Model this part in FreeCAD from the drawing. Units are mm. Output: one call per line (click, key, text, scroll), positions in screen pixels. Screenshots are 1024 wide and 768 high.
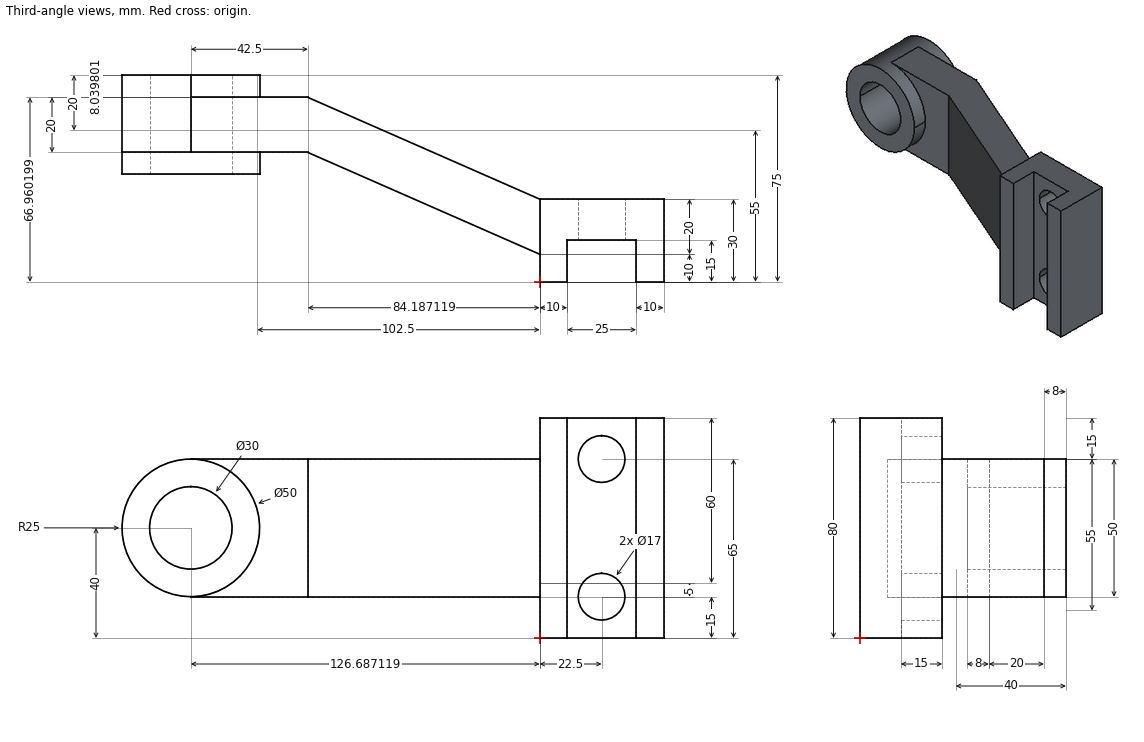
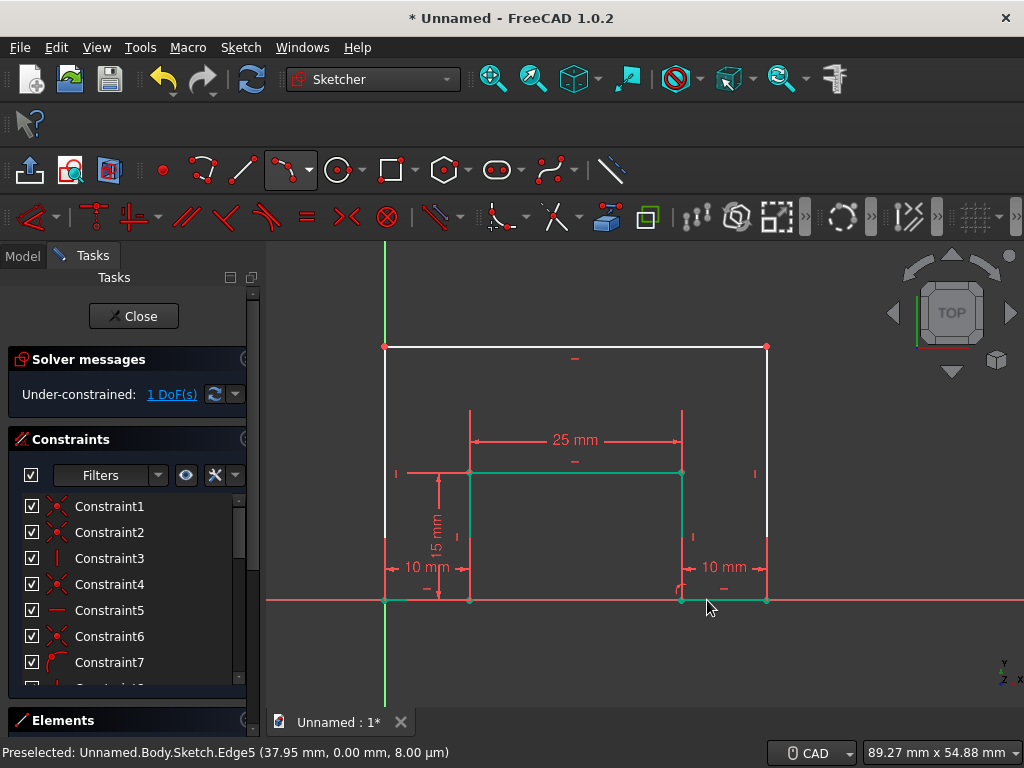
click(767, 524)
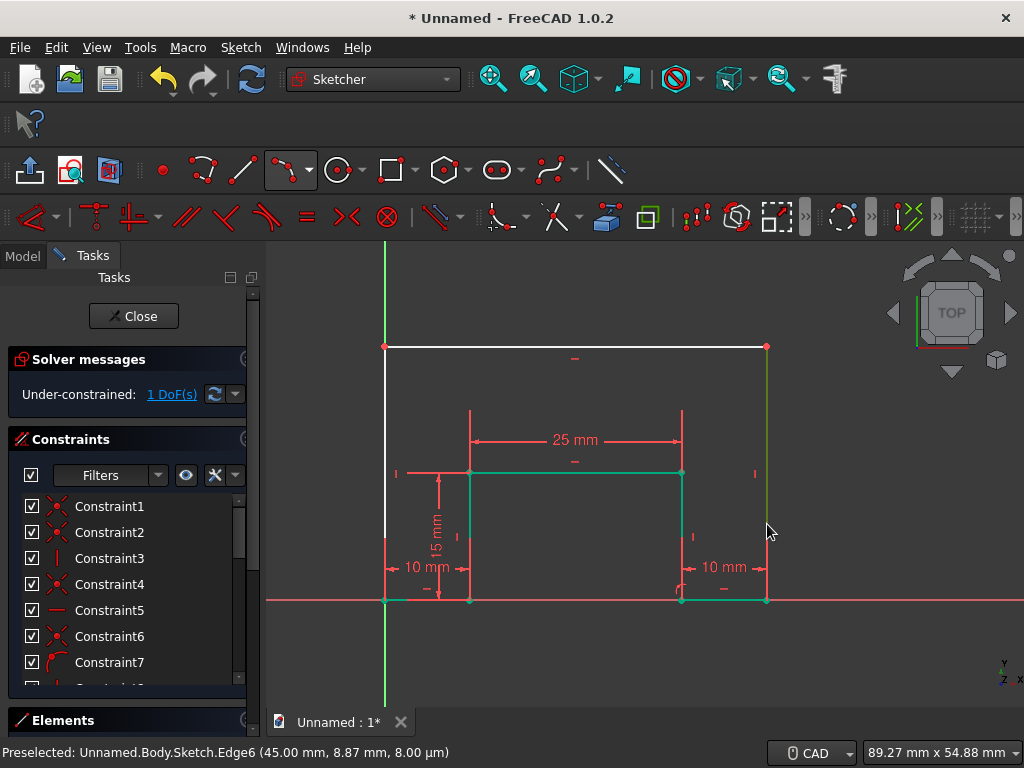
click(58, 218)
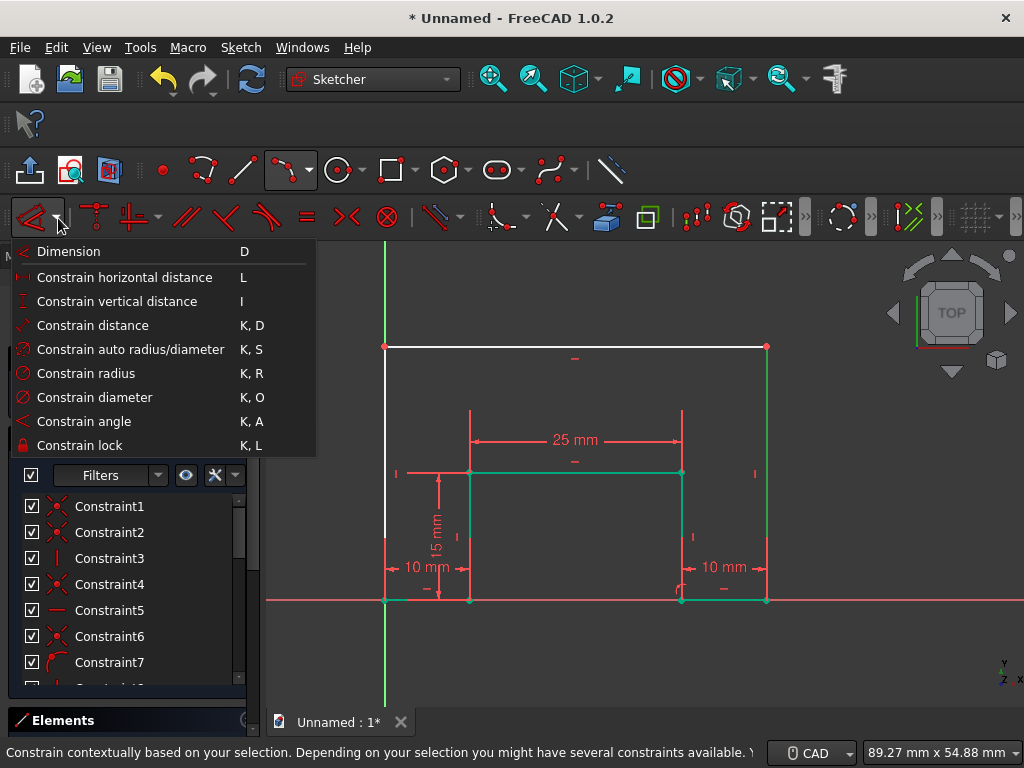
click(164, 301)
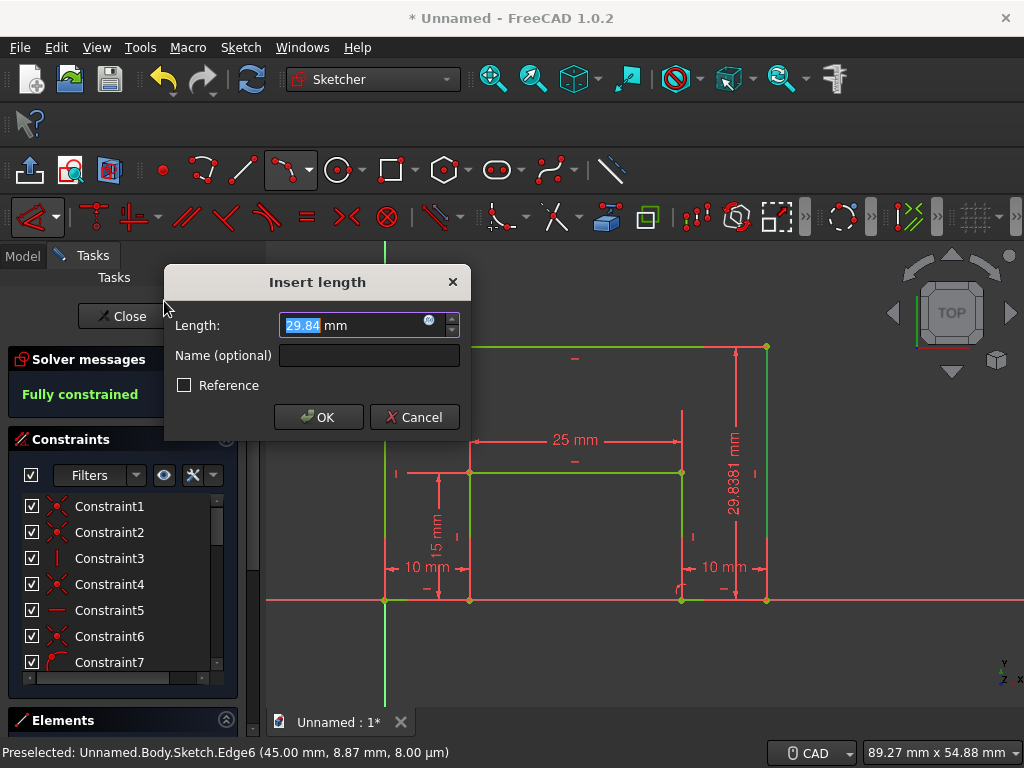
text(30)
key(Return)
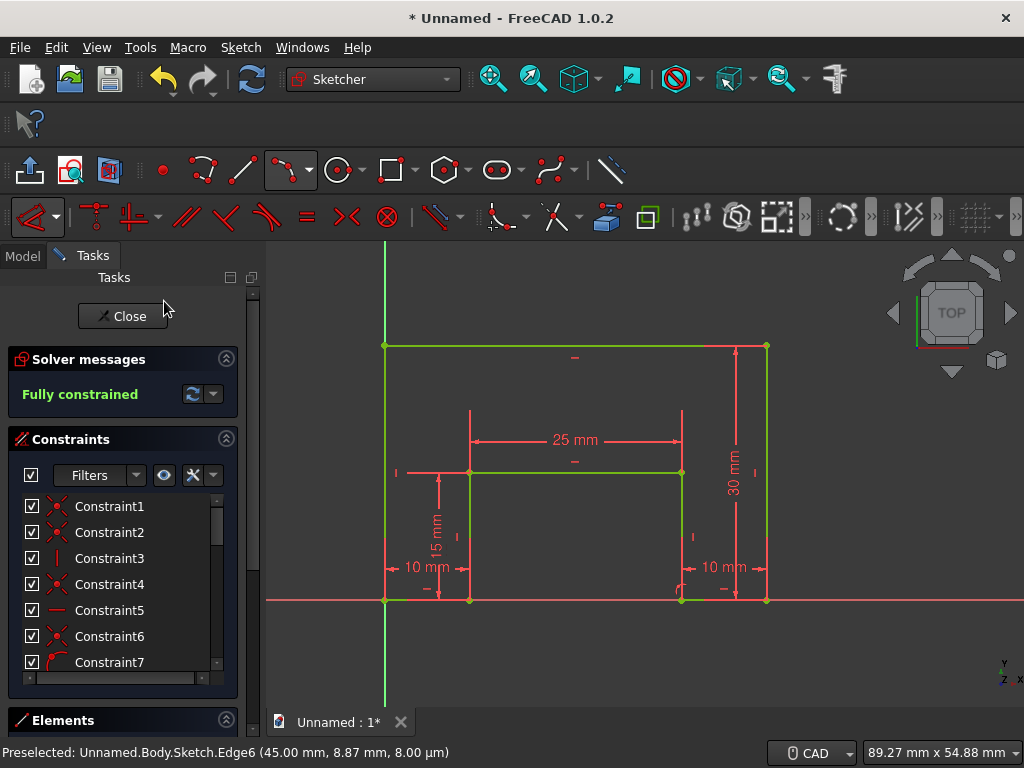
click(123, 316)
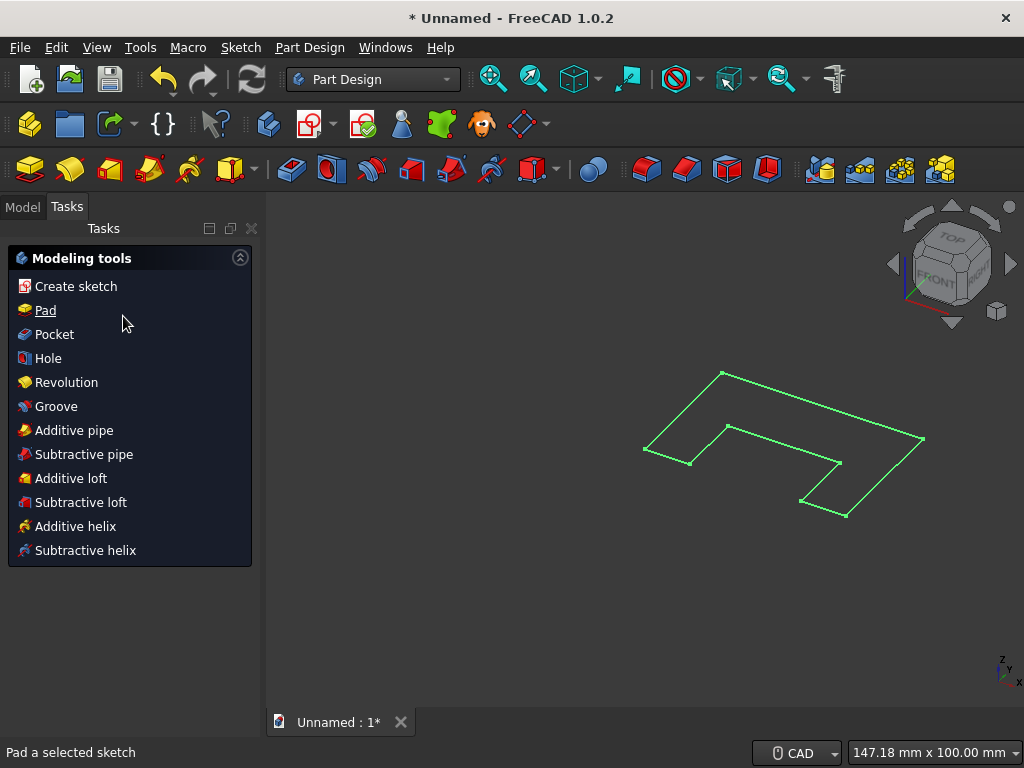
click(30, 170)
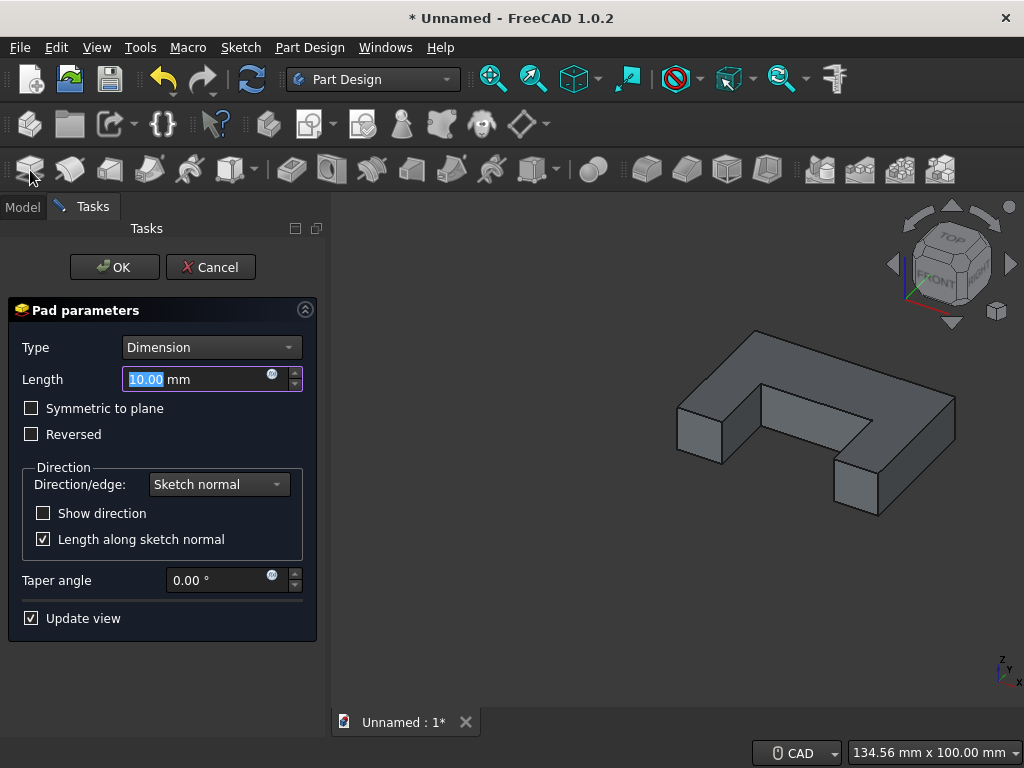
text(80)
key(Tab)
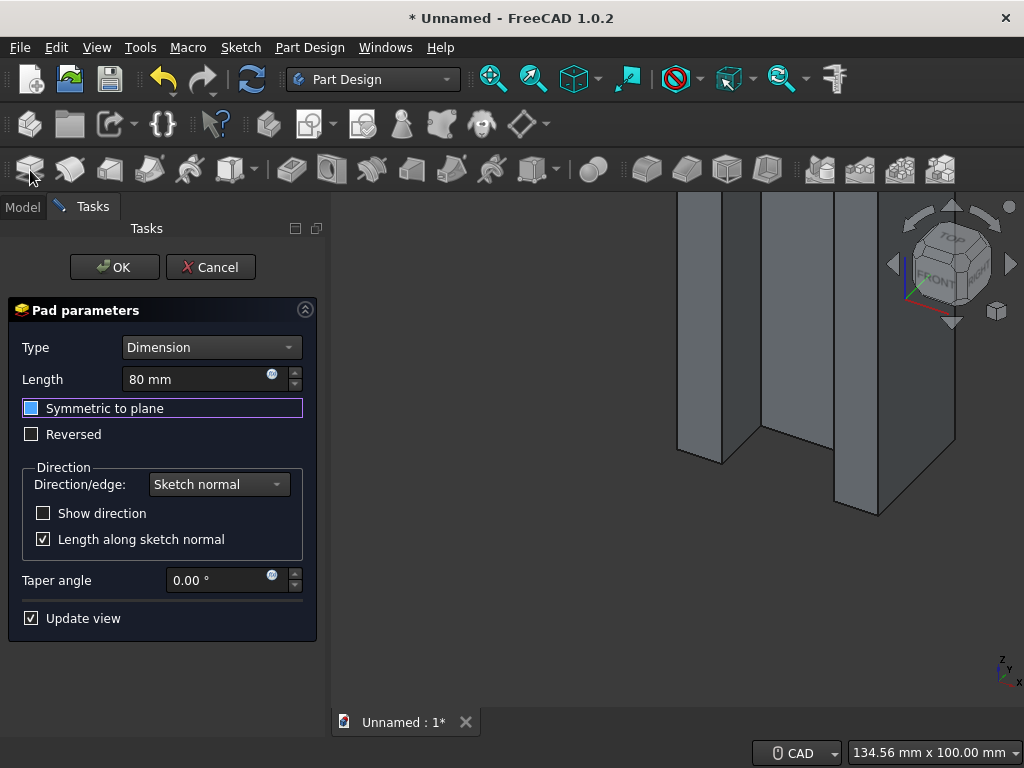
click(115, 267)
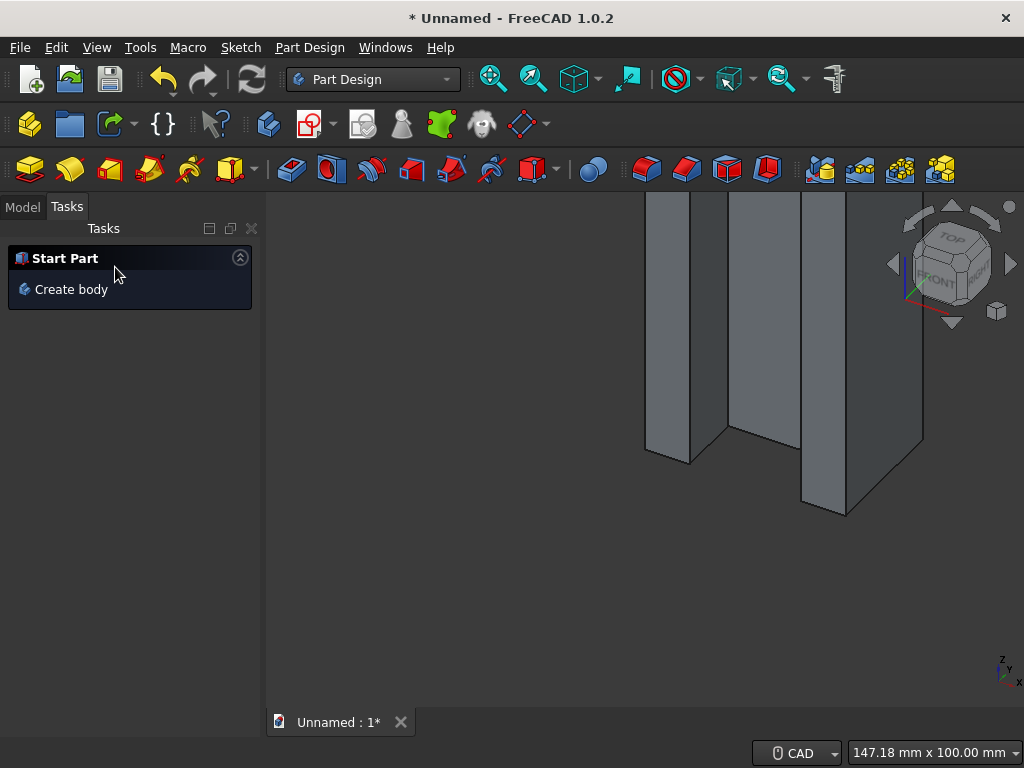
key(v)
key(f)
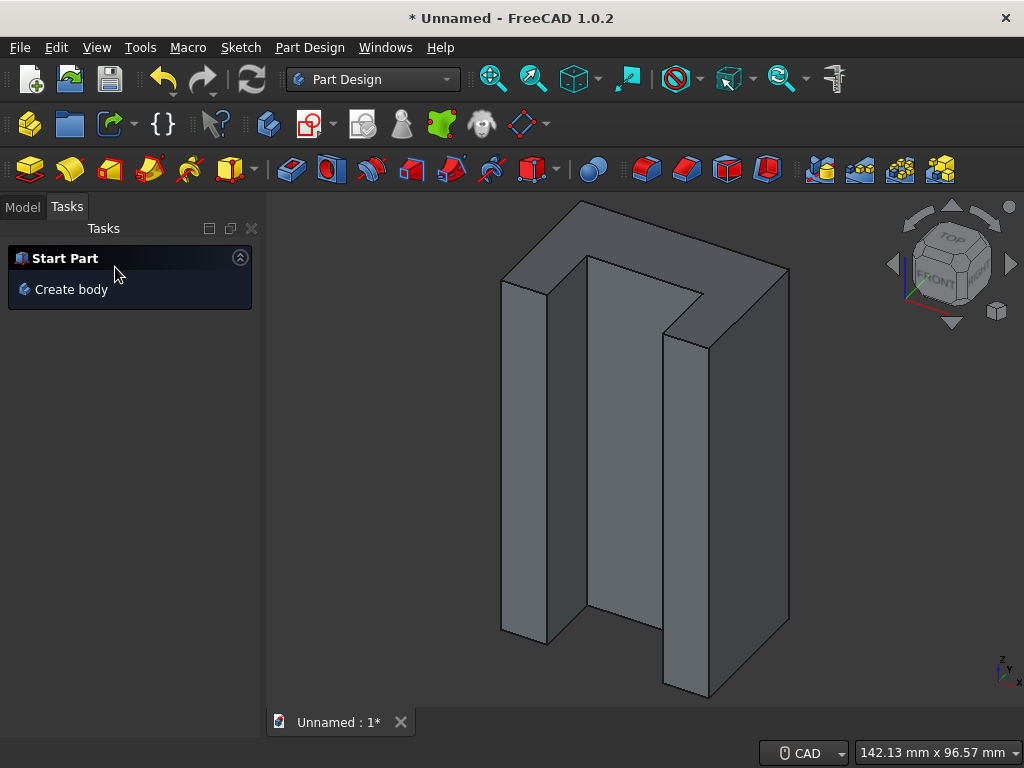
click(727, 271)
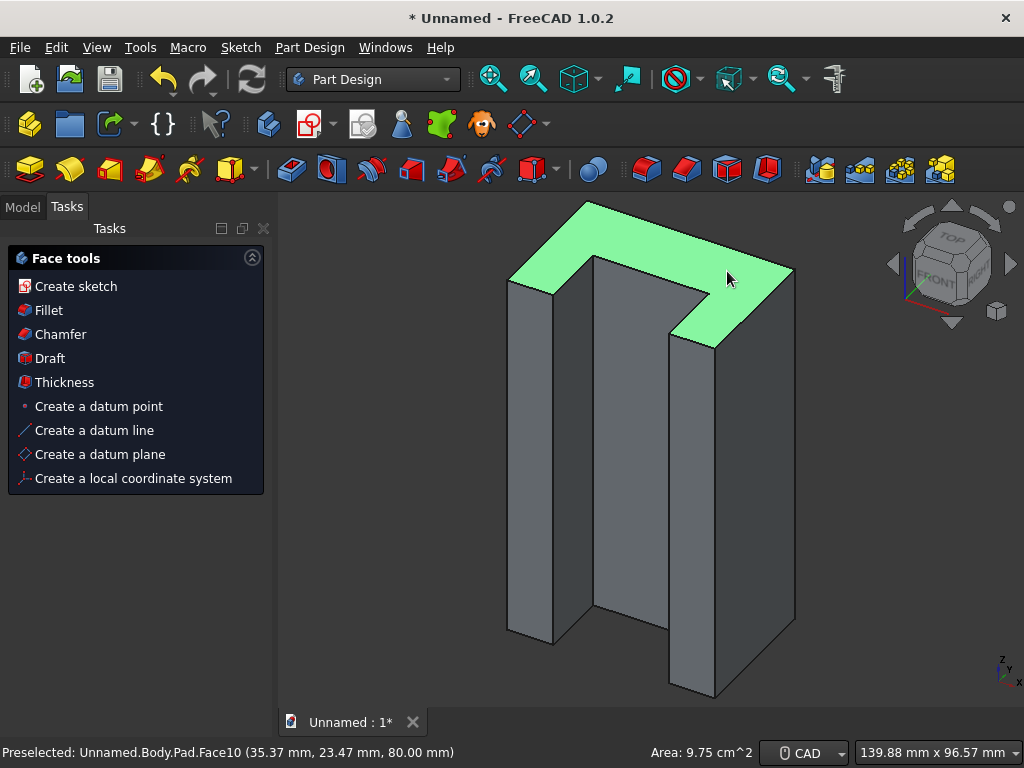
click(310, 124)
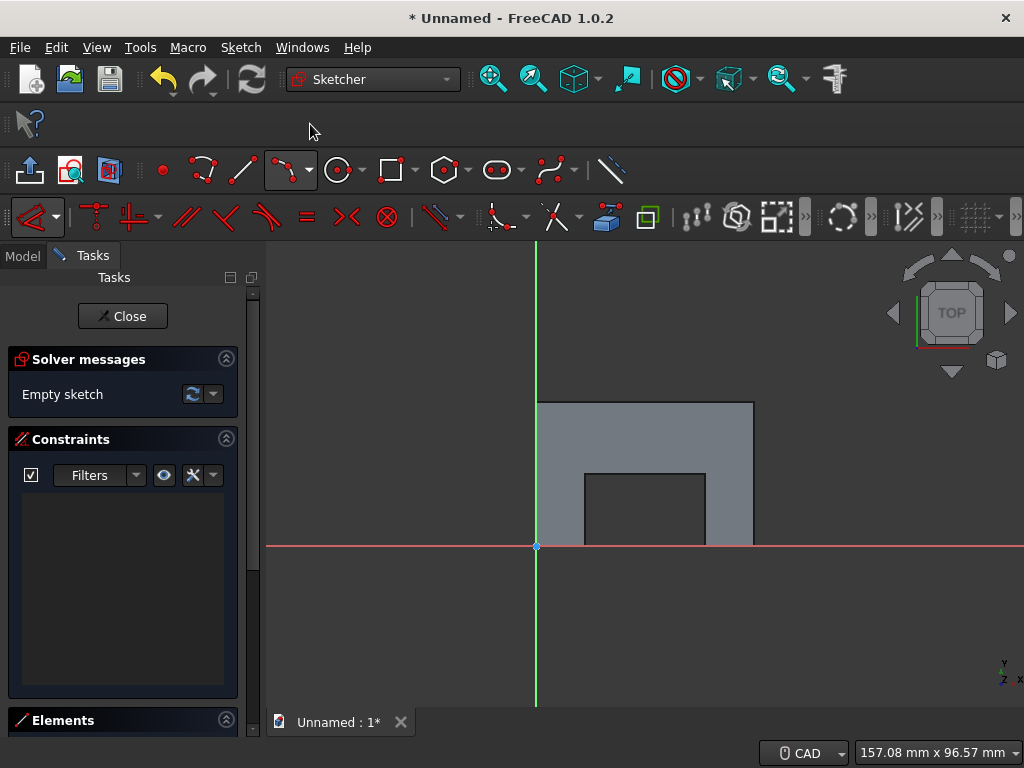
scroll(859, 606, down, 3)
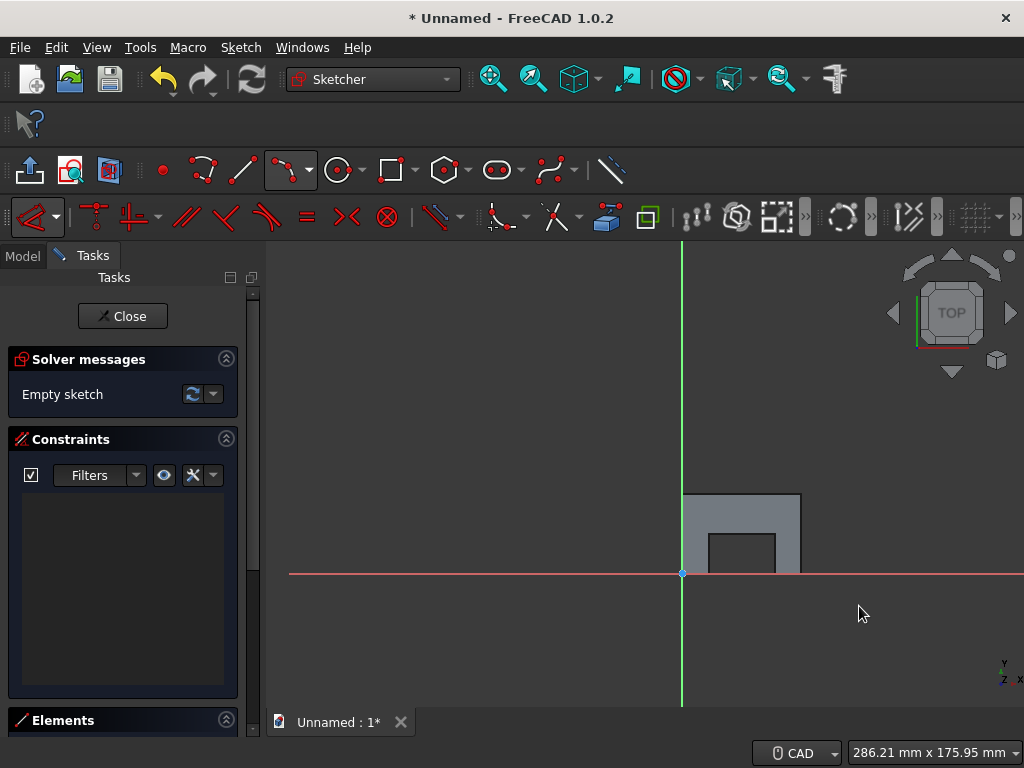
scroll(486, 475, up, 2)